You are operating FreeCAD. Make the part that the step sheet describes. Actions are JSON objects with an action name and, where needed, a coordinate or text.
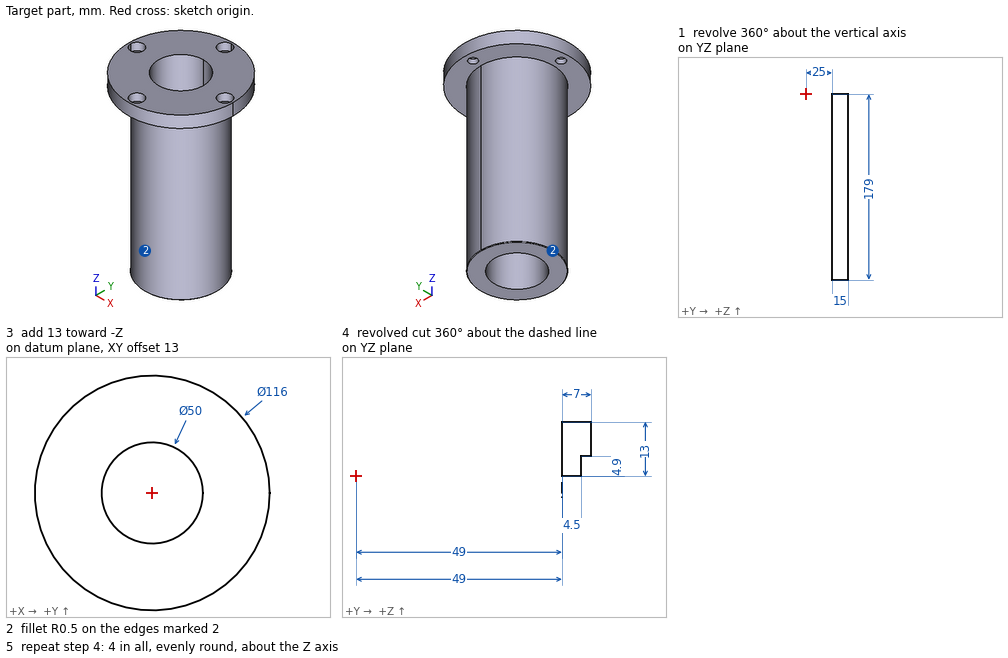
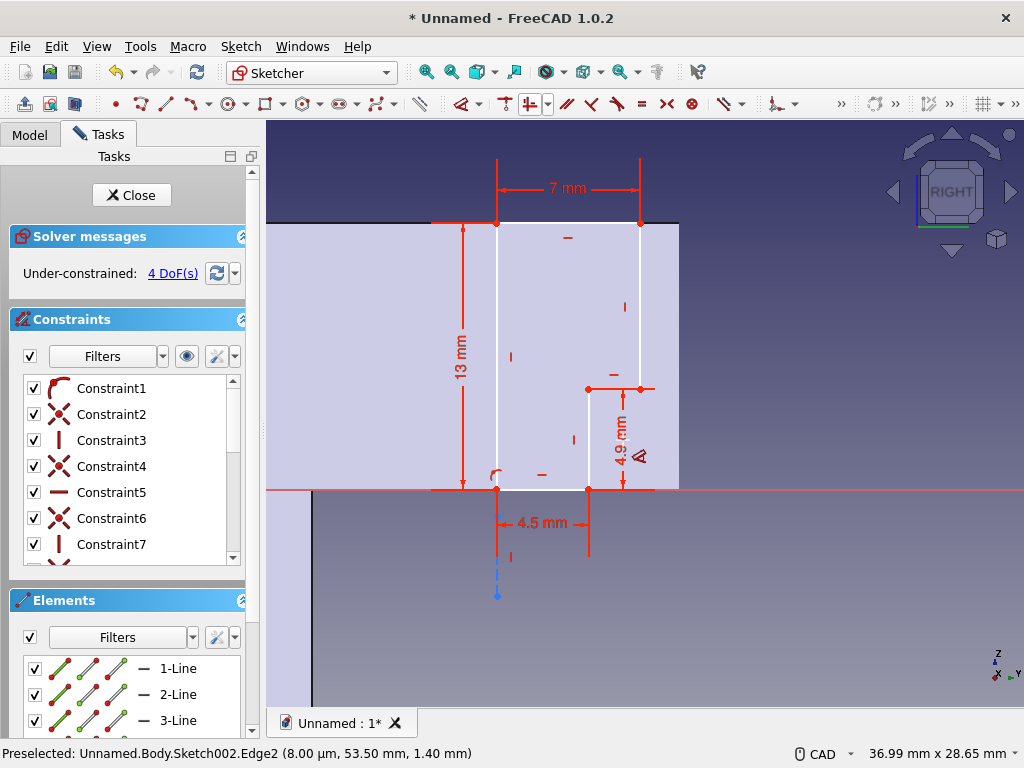
{"action": "left_click", "coordinate": [497, 490]}
{"action": "left_click", "coordinate": [395, 524]}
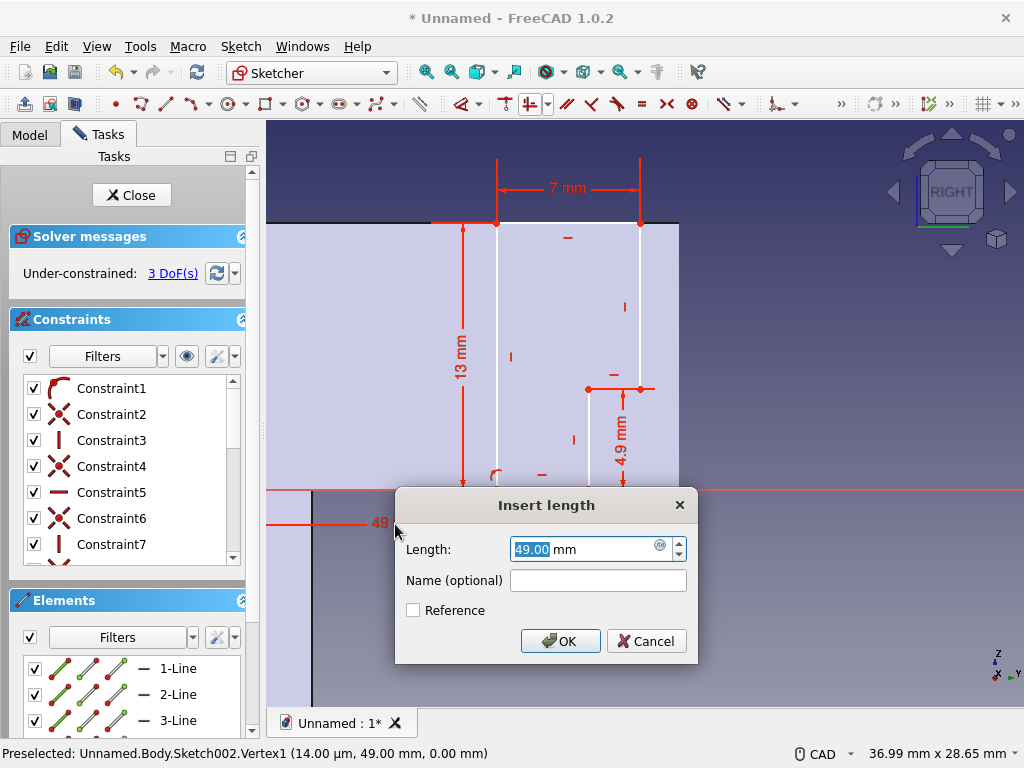
{"action": "type", "text": "49"}
{"action": "key", "text": "Return"}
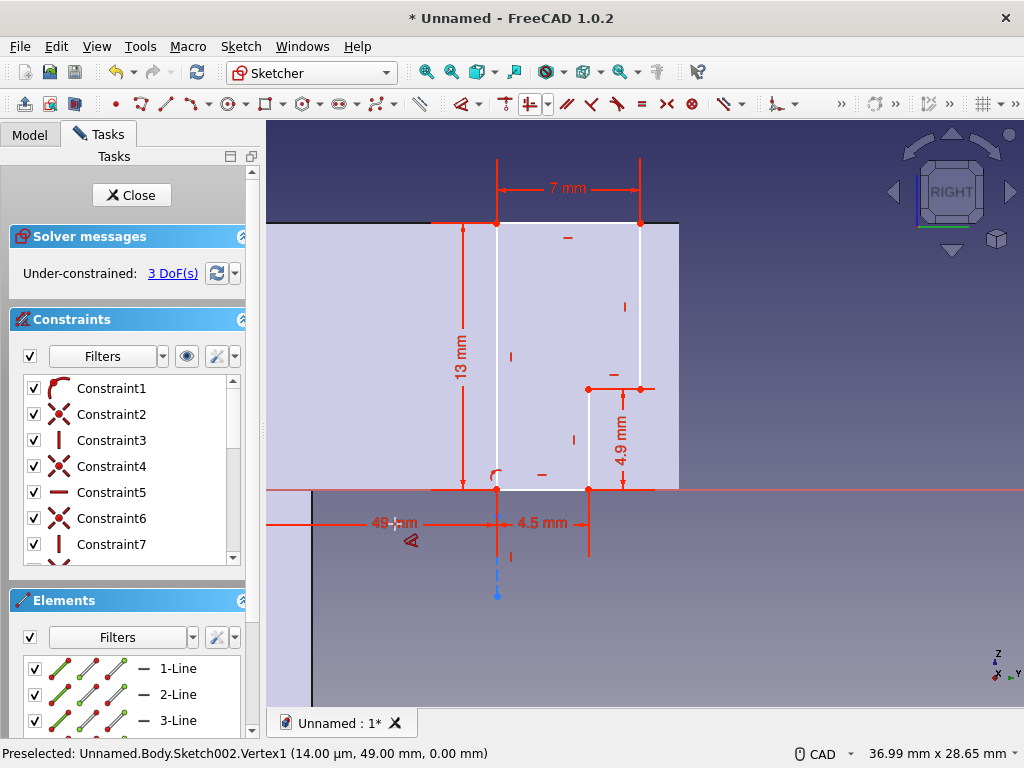
{"action": "left_click", "coordinate": [497, 517]}
{"action": "left_click", "coordinate": [396, 551]}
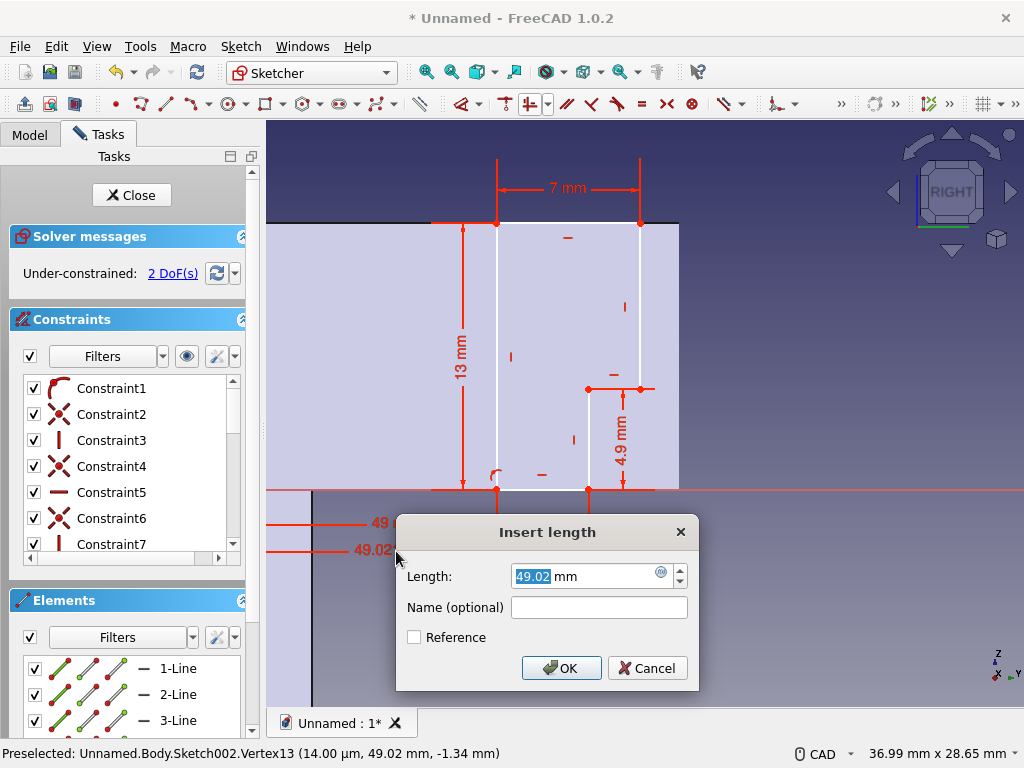
{"action": "type", "text": "49"}
{"action": "key", "text": "Return"}
{"action": "key", "text": "Escape"}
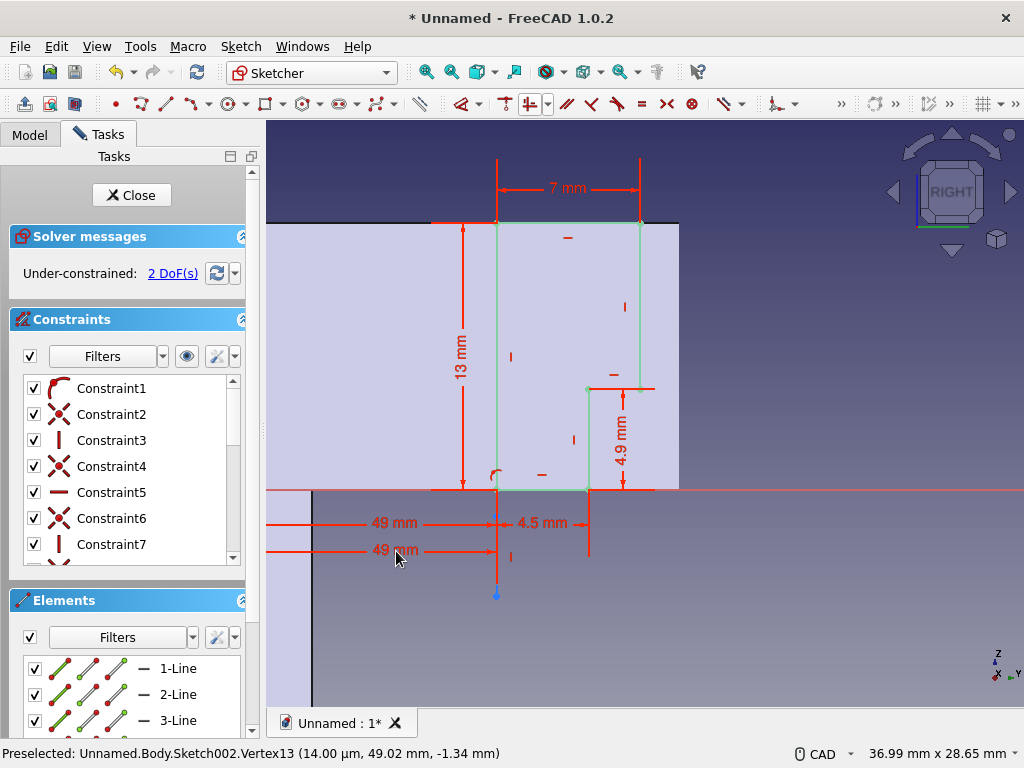
{"action": "left_click", "coordinate": [132, 195]}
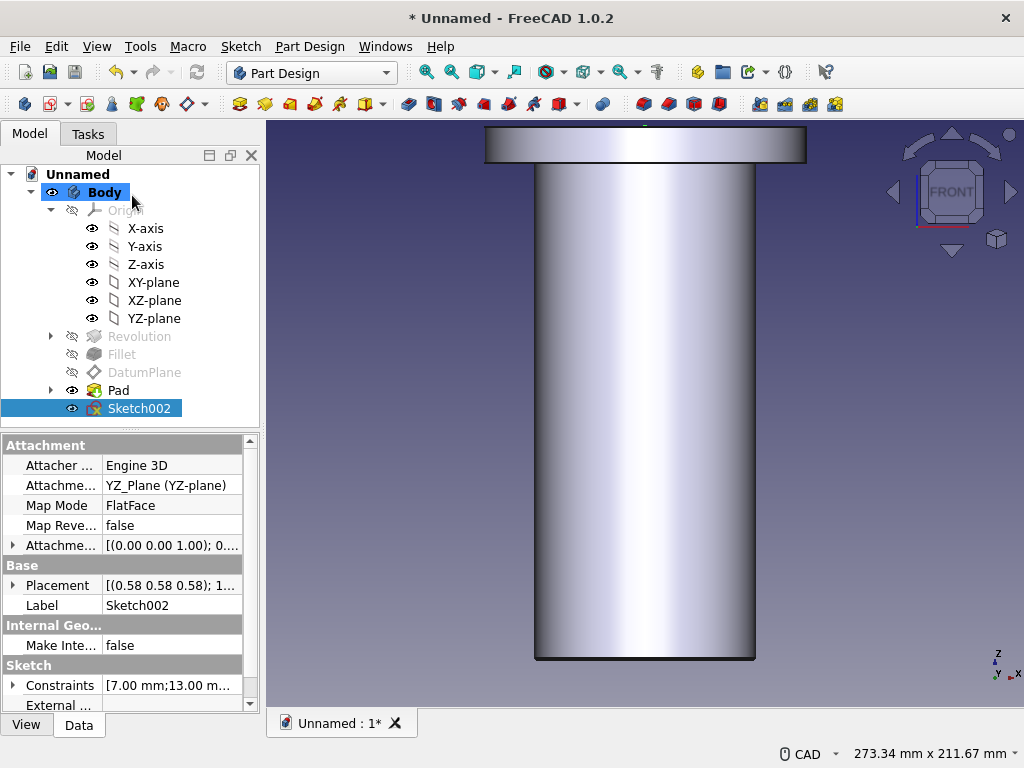
{"action": "left_click", "coordinate": [459, 104]}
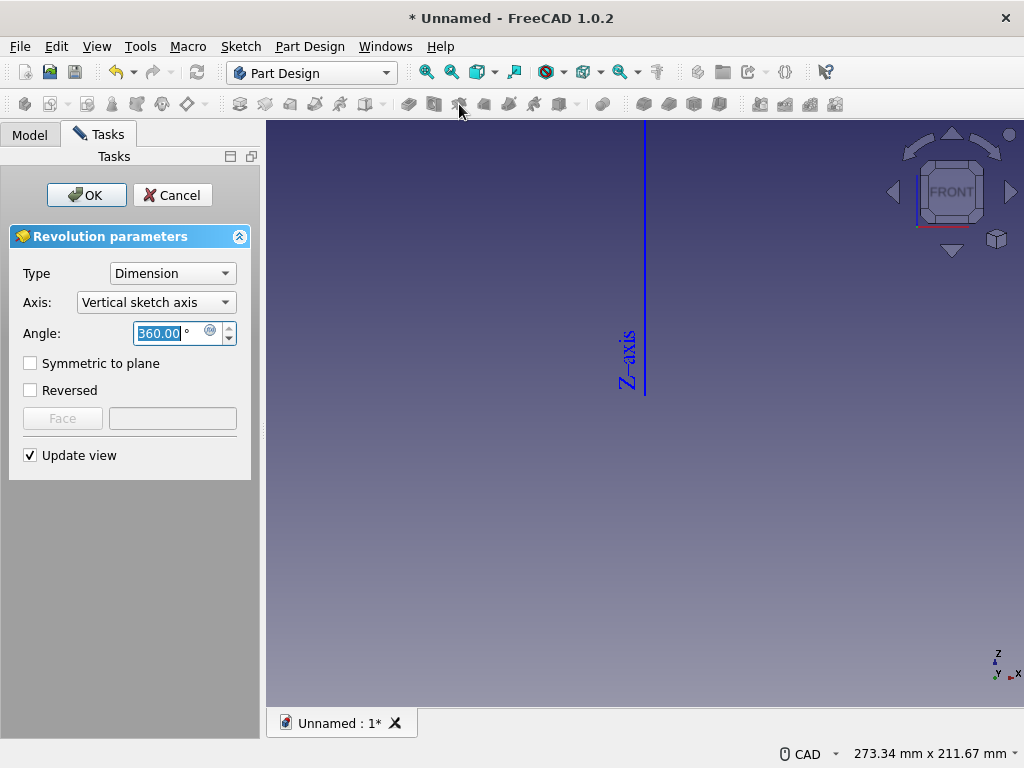
{"action": "left_click", "coordinate": [157, 302]}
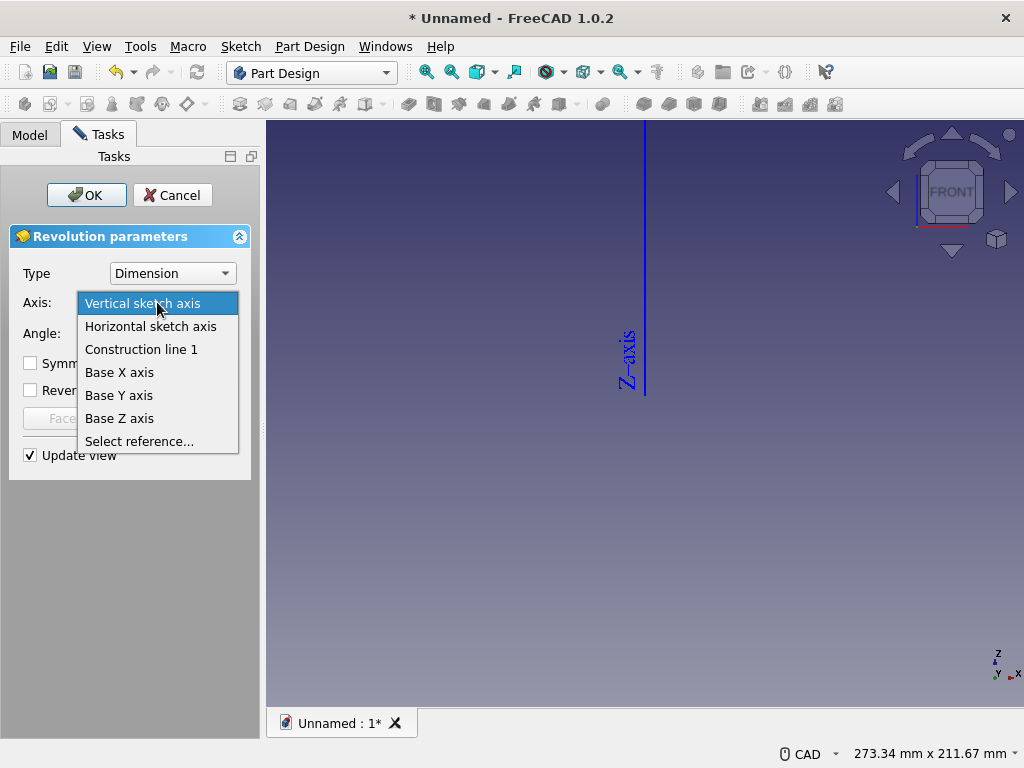
{"action": "left_click", "coordinate": [156, 350]}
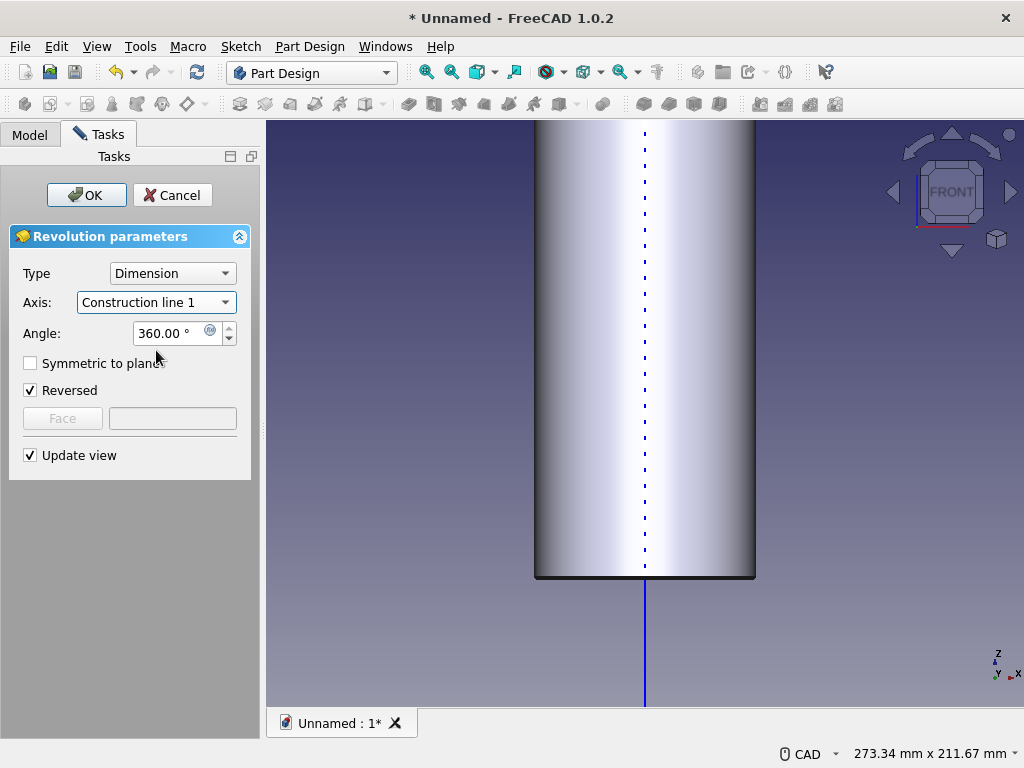
{"action": "left_click", "coordinate": [87, 195]}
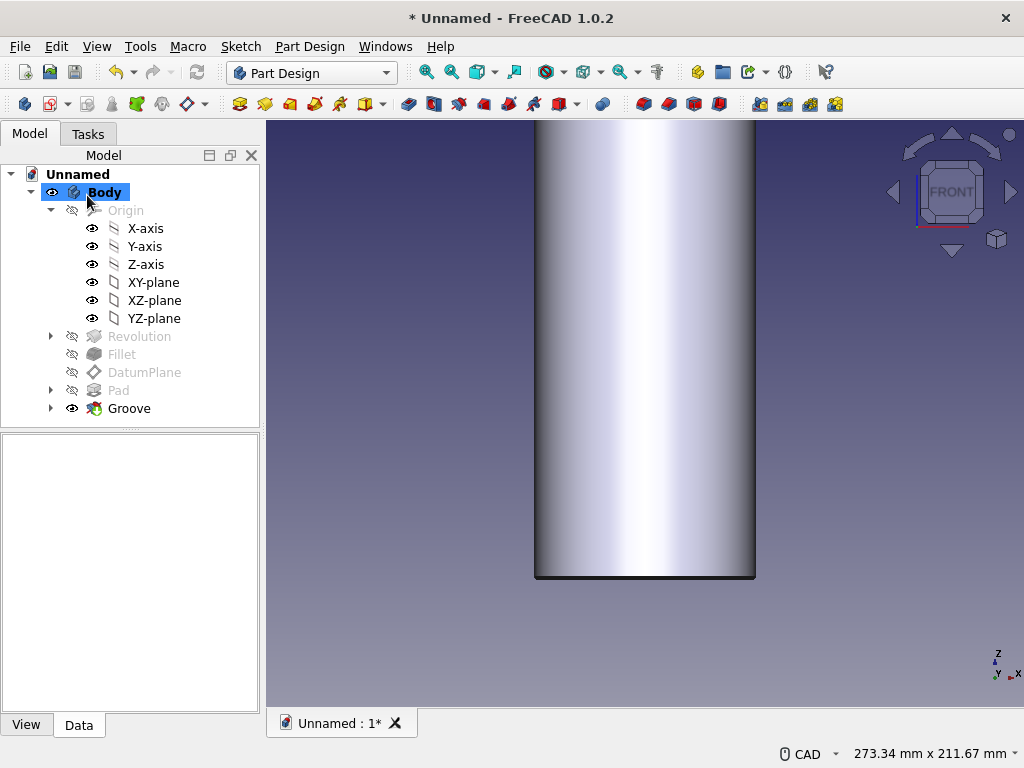
{"action": "left_click", "coordinate": [427, 72]}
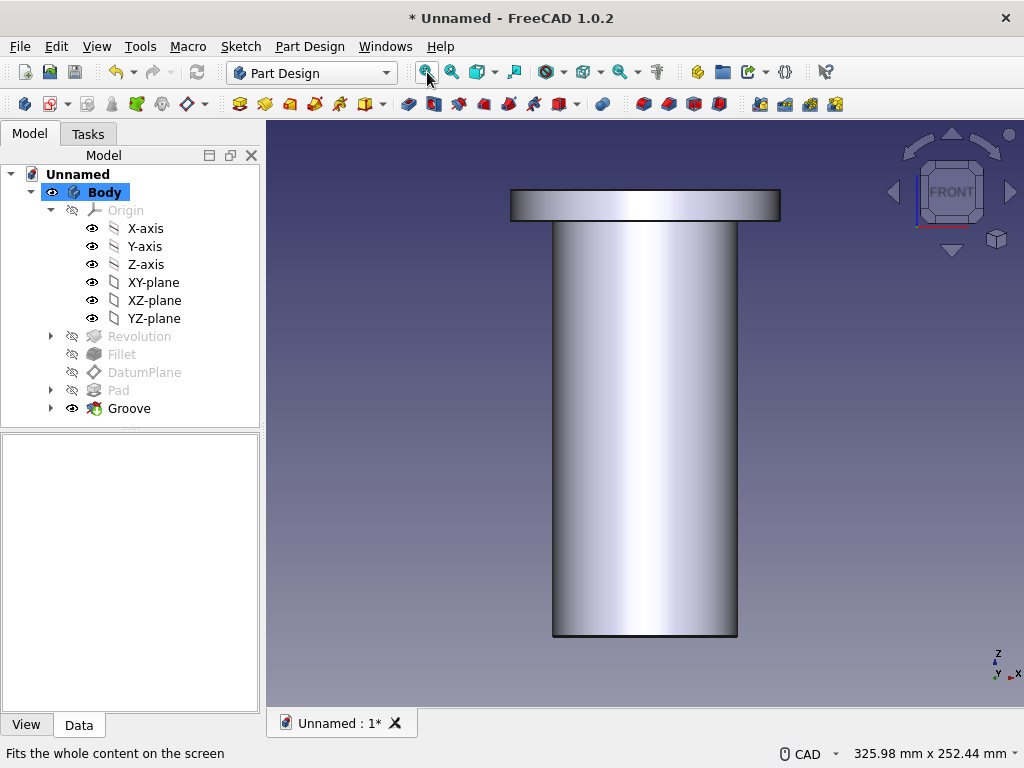
{"action": "left_click", "coordinate": [117, 408]}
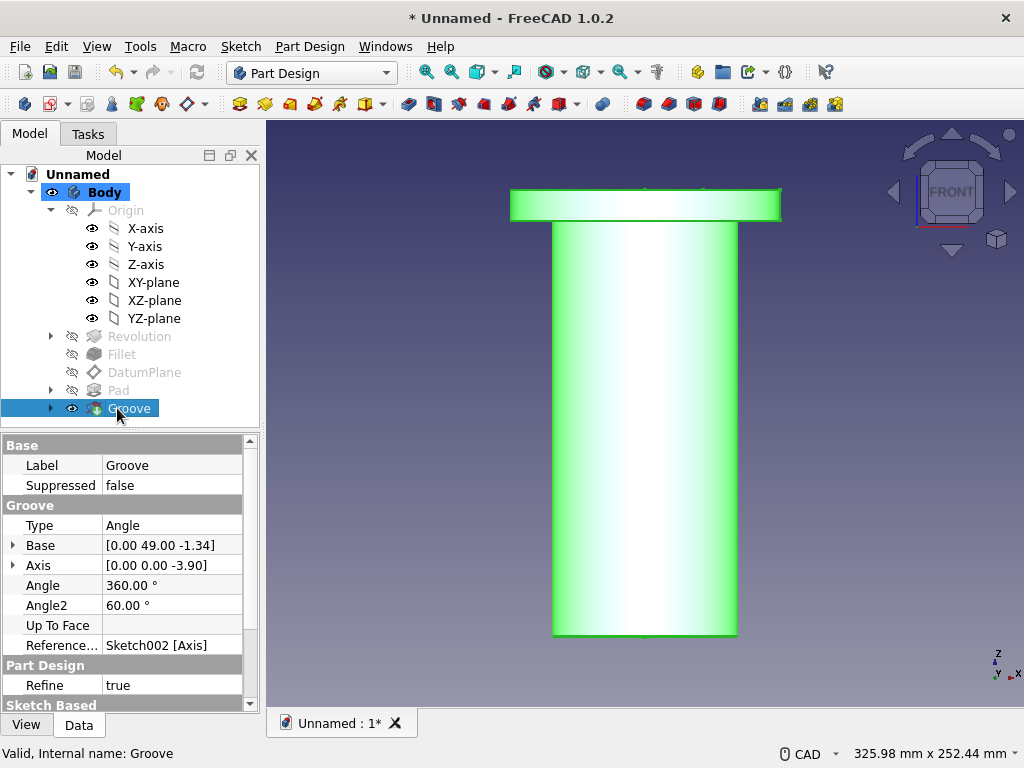
{"action": "left_click", "coordinate": [810, 104]}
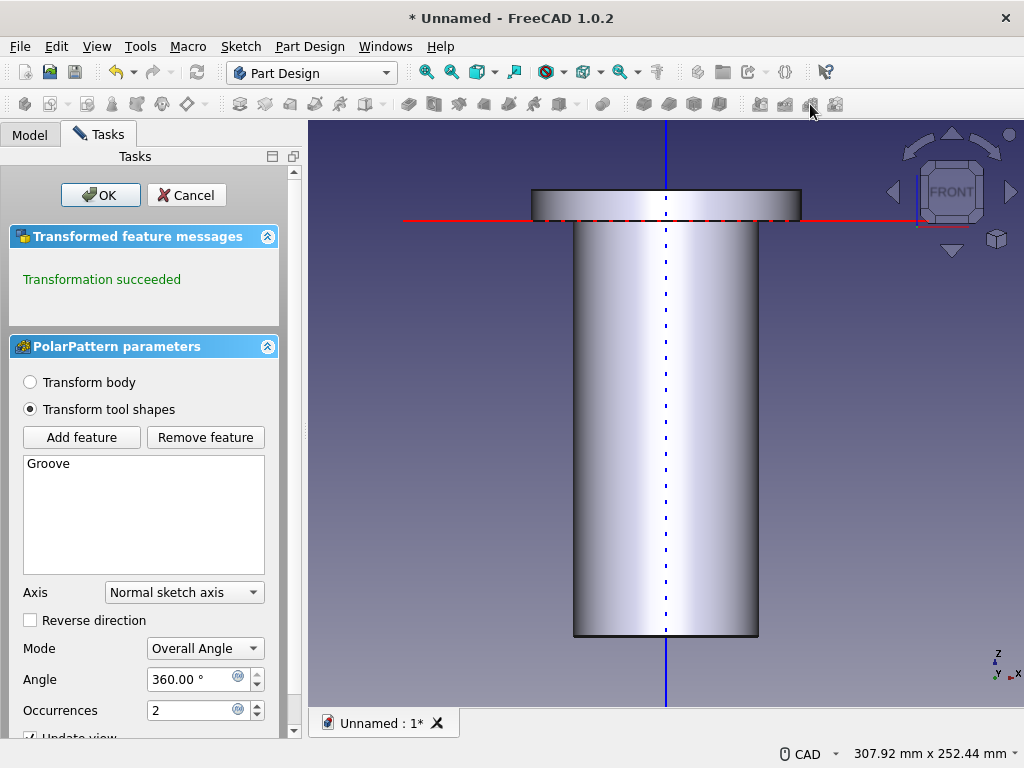
{"action": "left_click", "coordinate": [185, 592]}